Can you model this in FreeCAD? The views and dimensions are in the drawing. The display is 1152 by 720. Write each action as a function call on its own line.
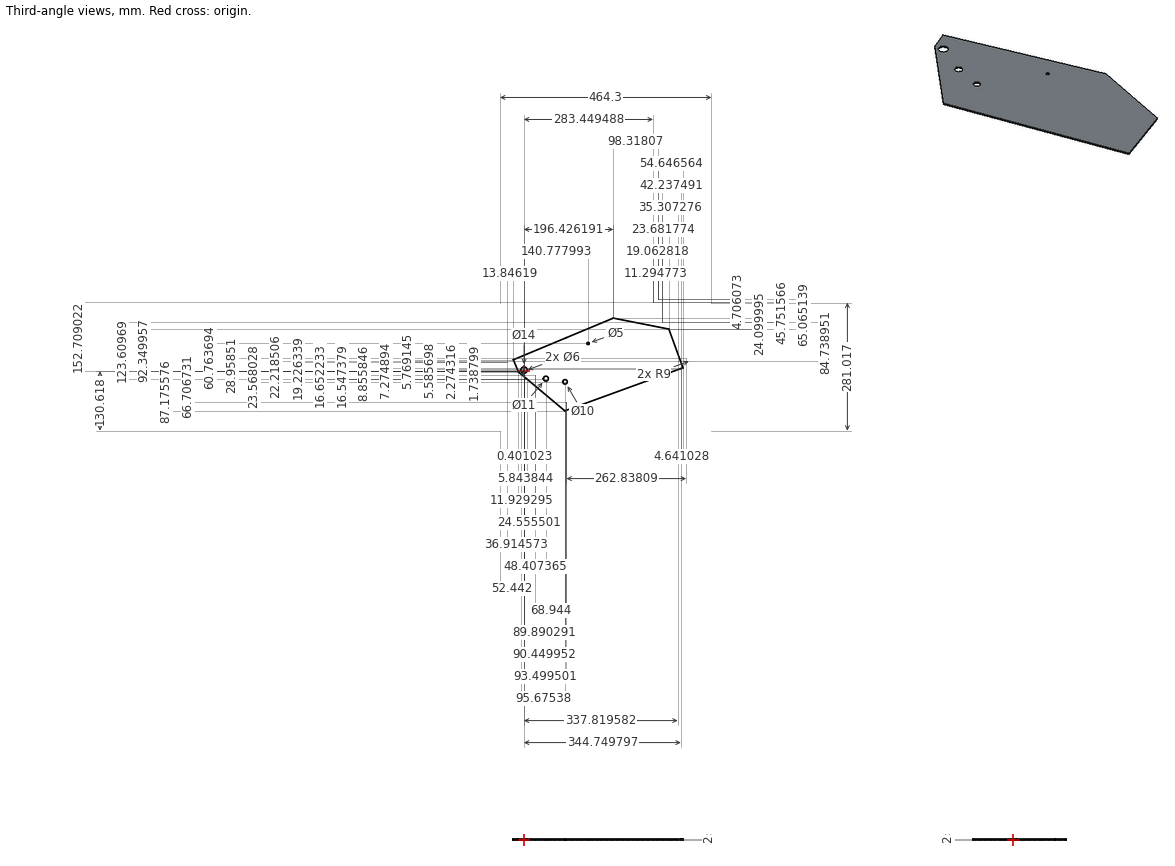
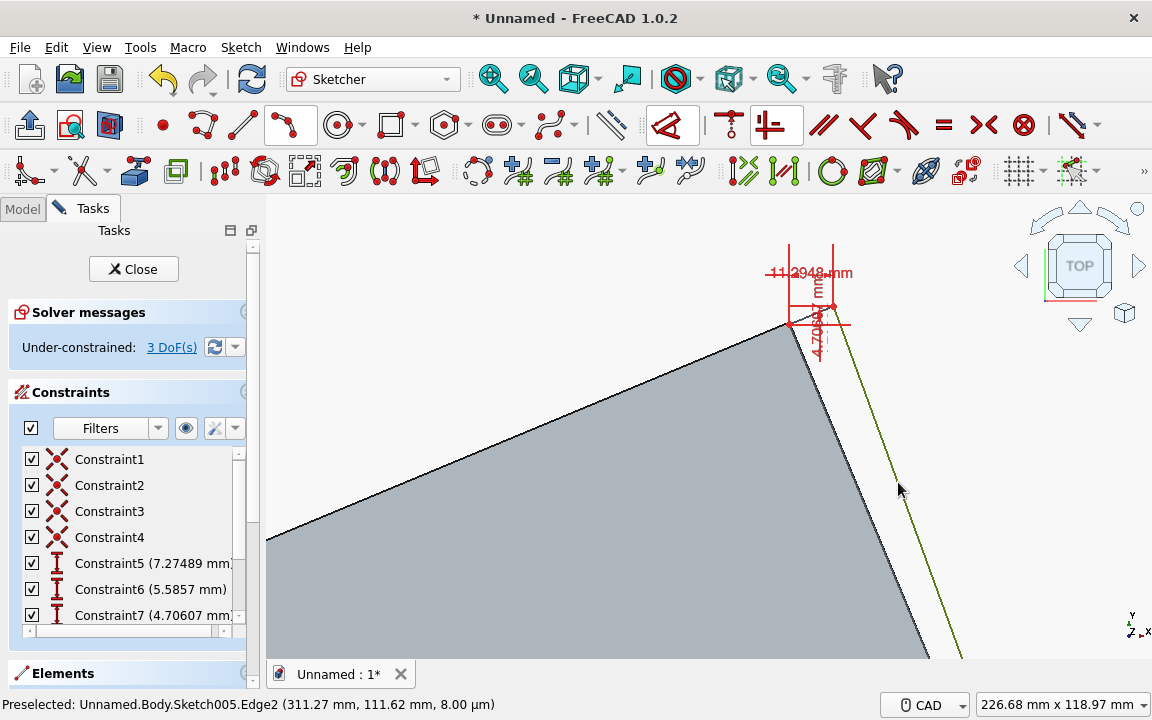
key(l)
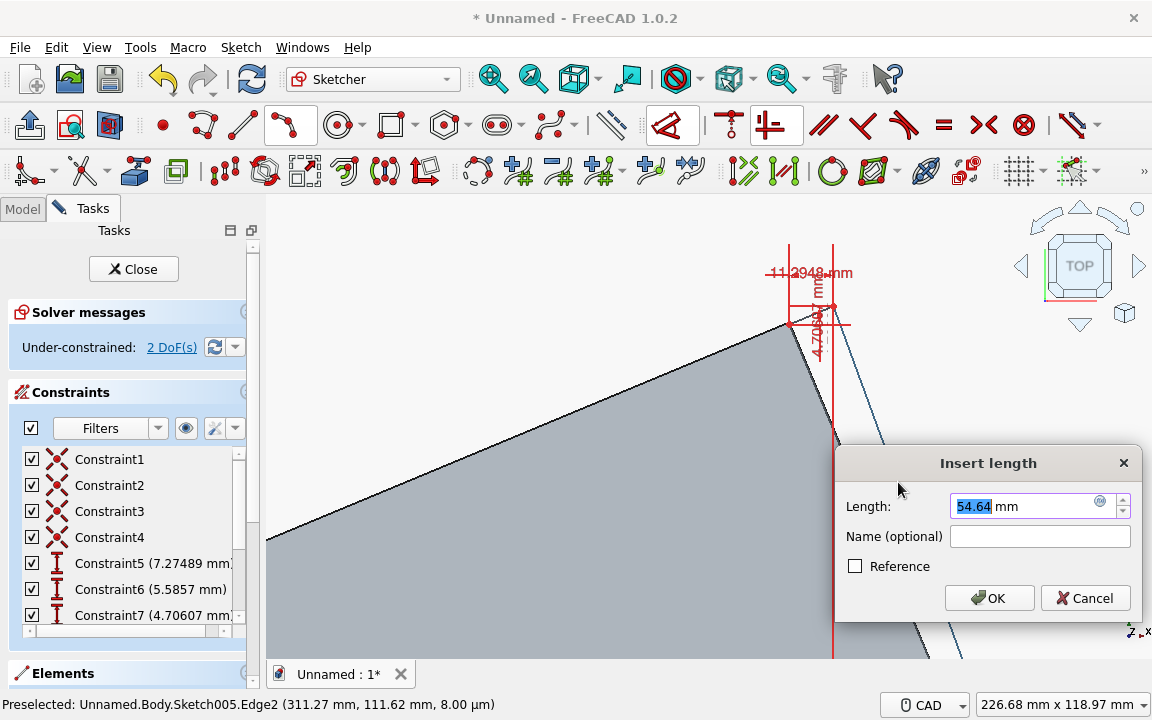
text(54.646564)
key(Return)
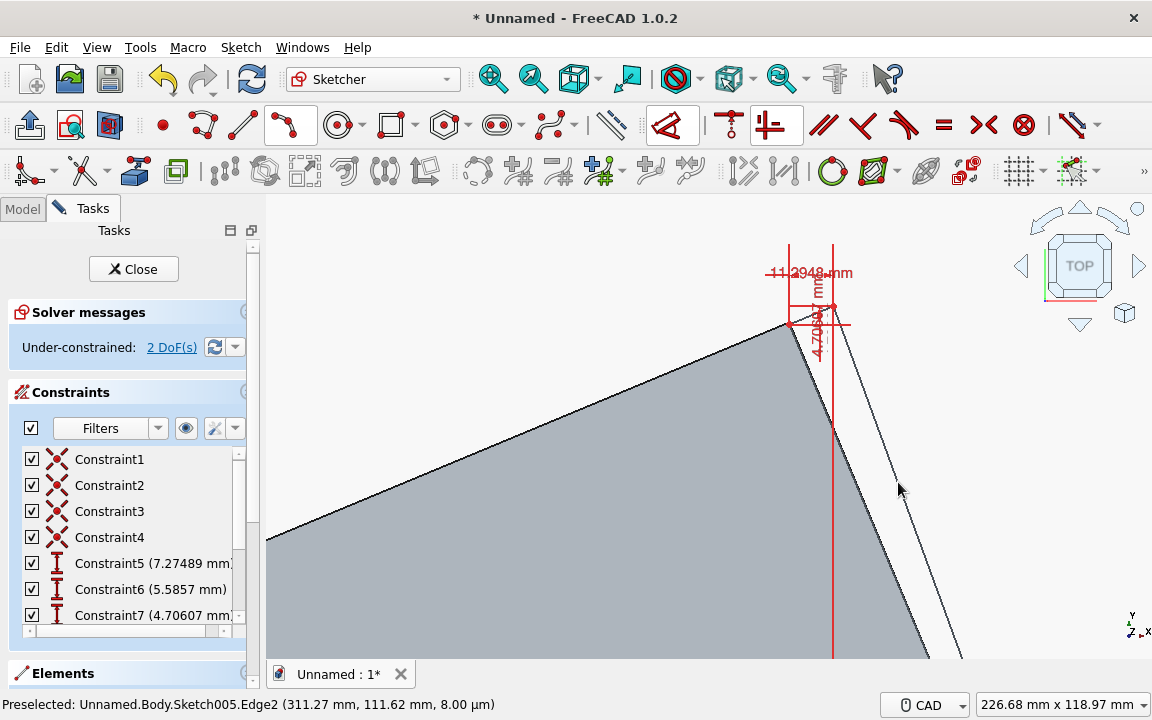
click(789, 325)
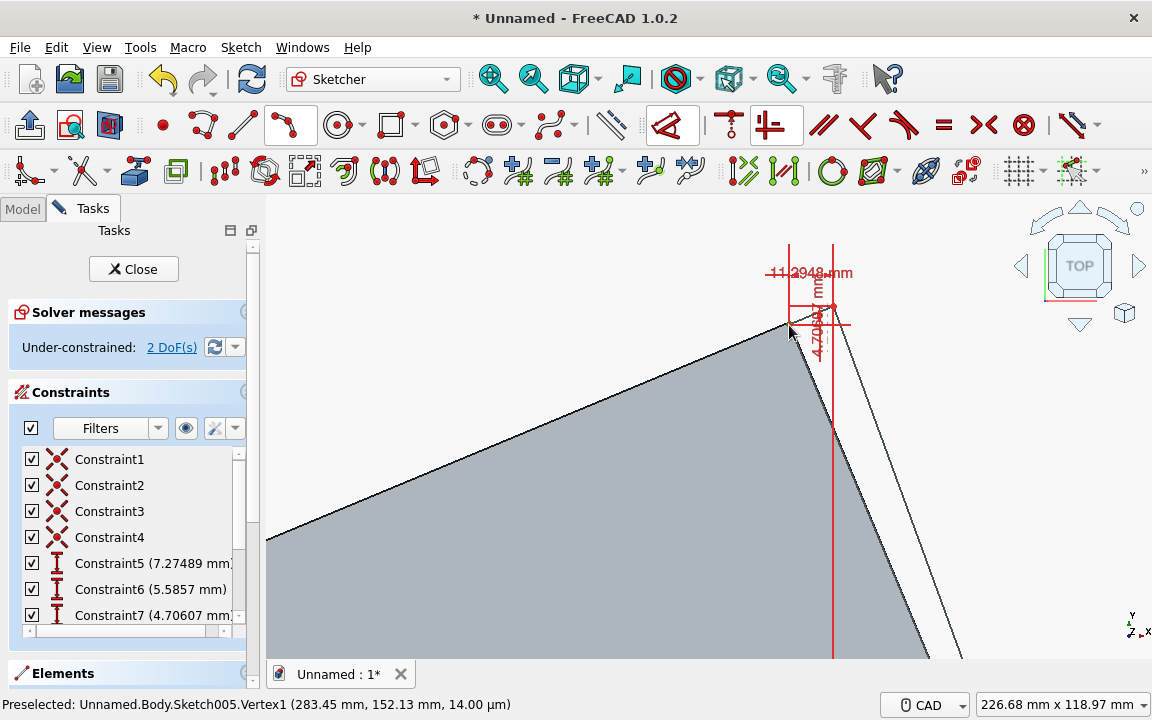
key(l)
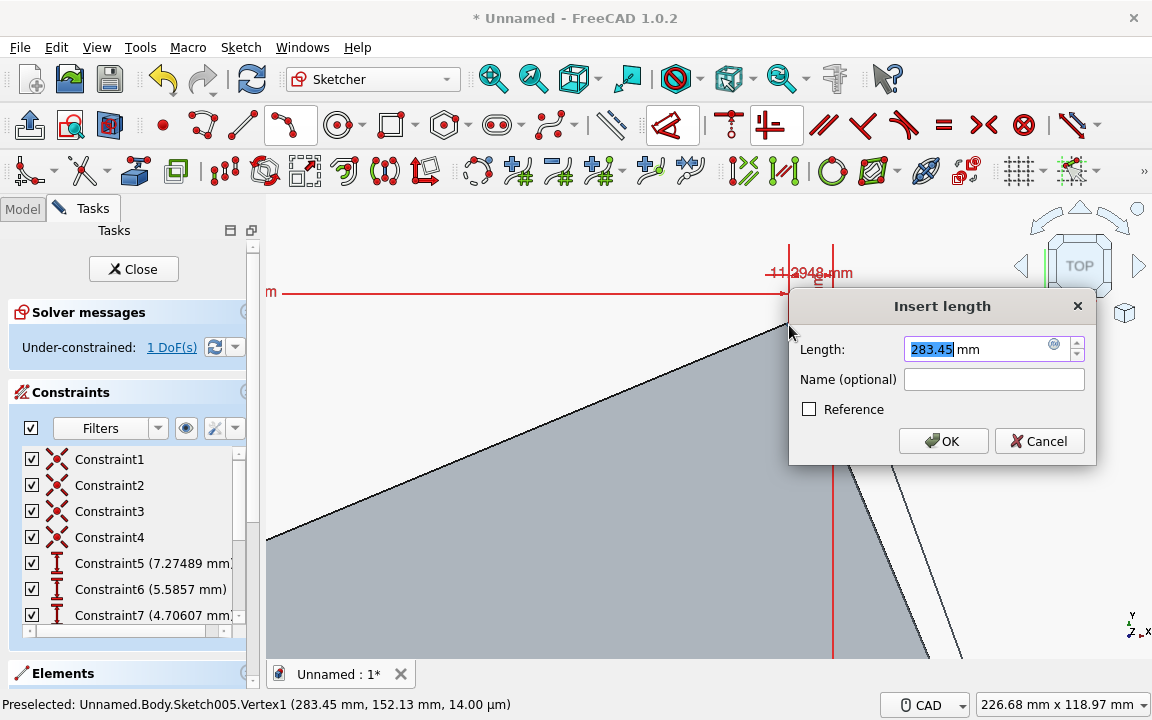
text(283.449488)
key(Return)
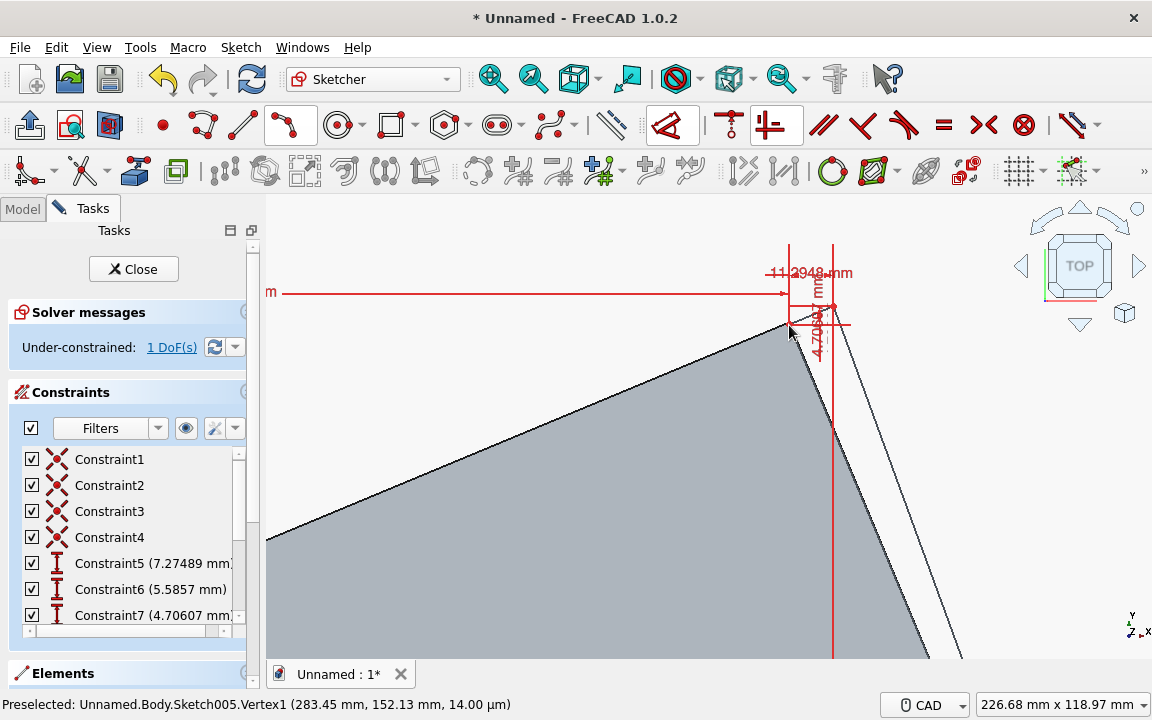
click(789, 325)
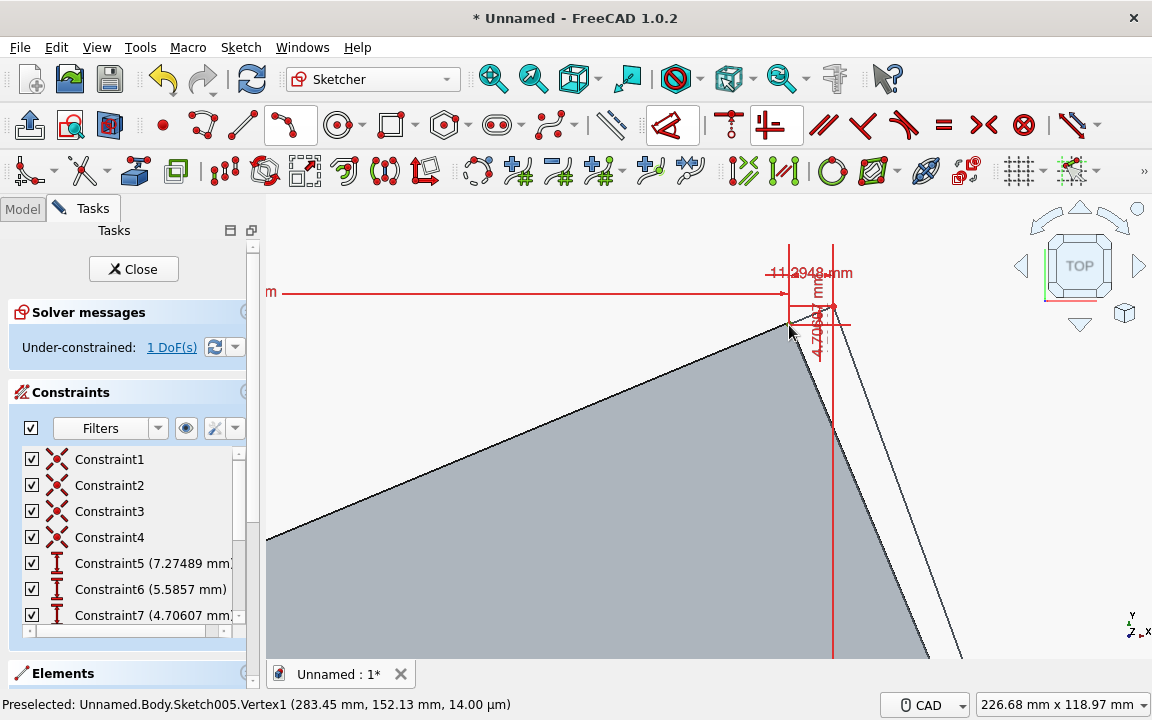
key(i)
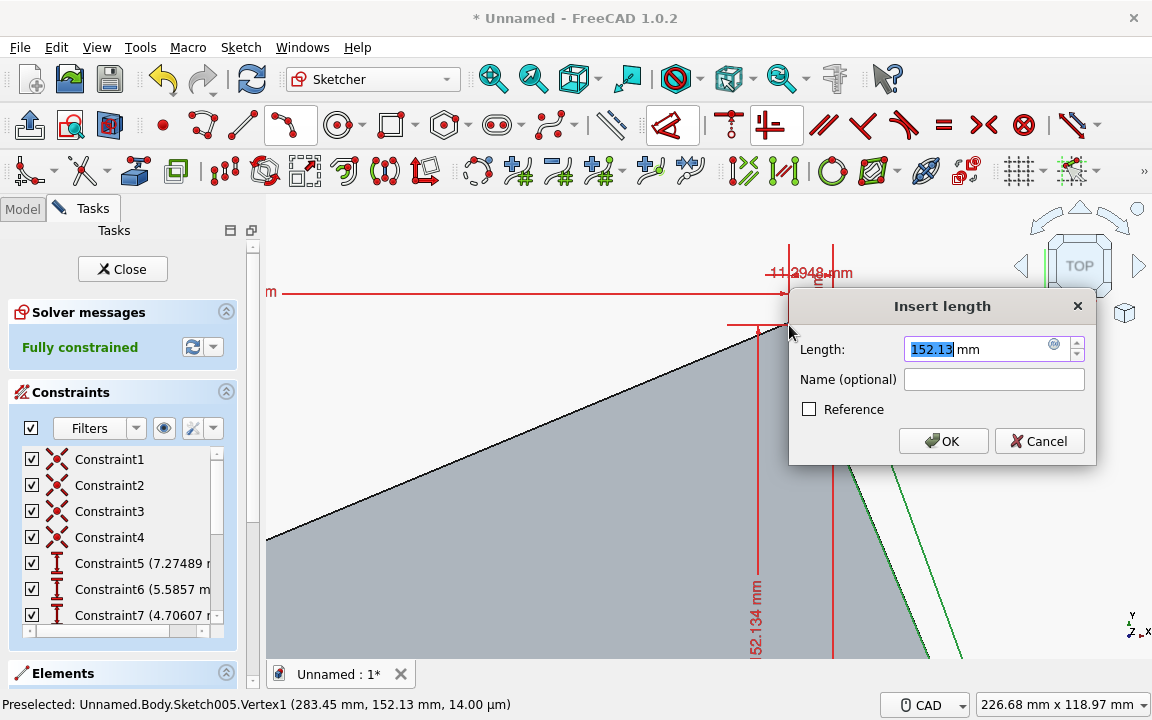
text(152.709022)
key(Return)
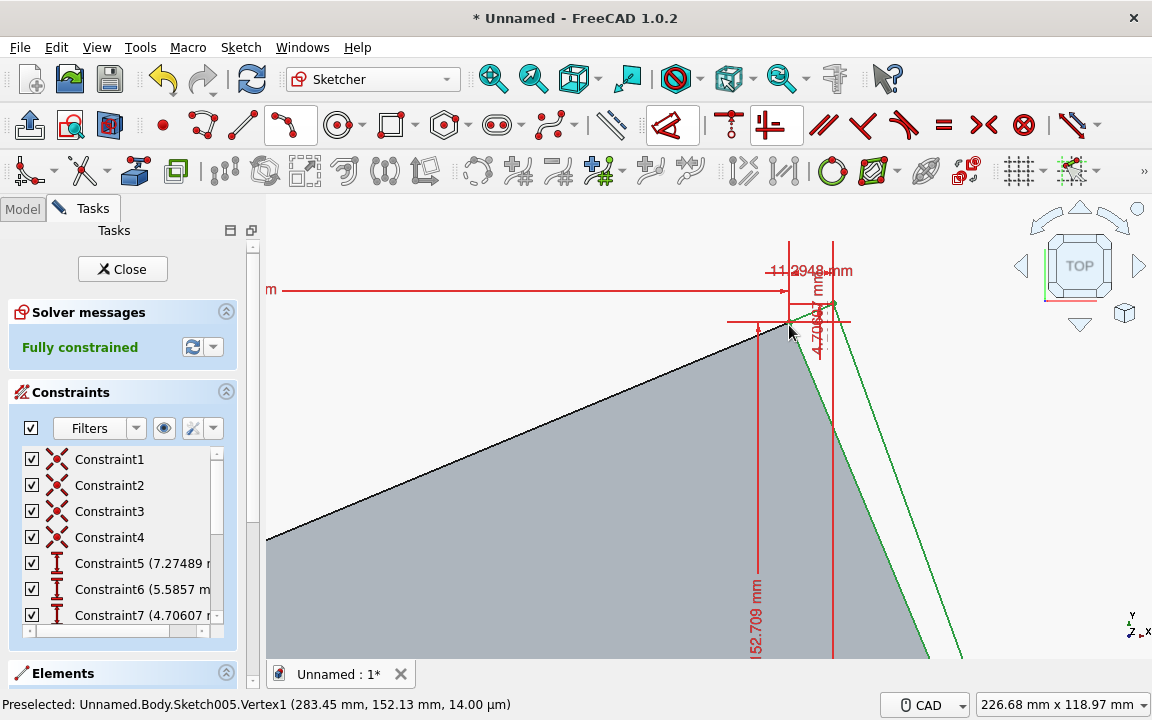
click(123, 269)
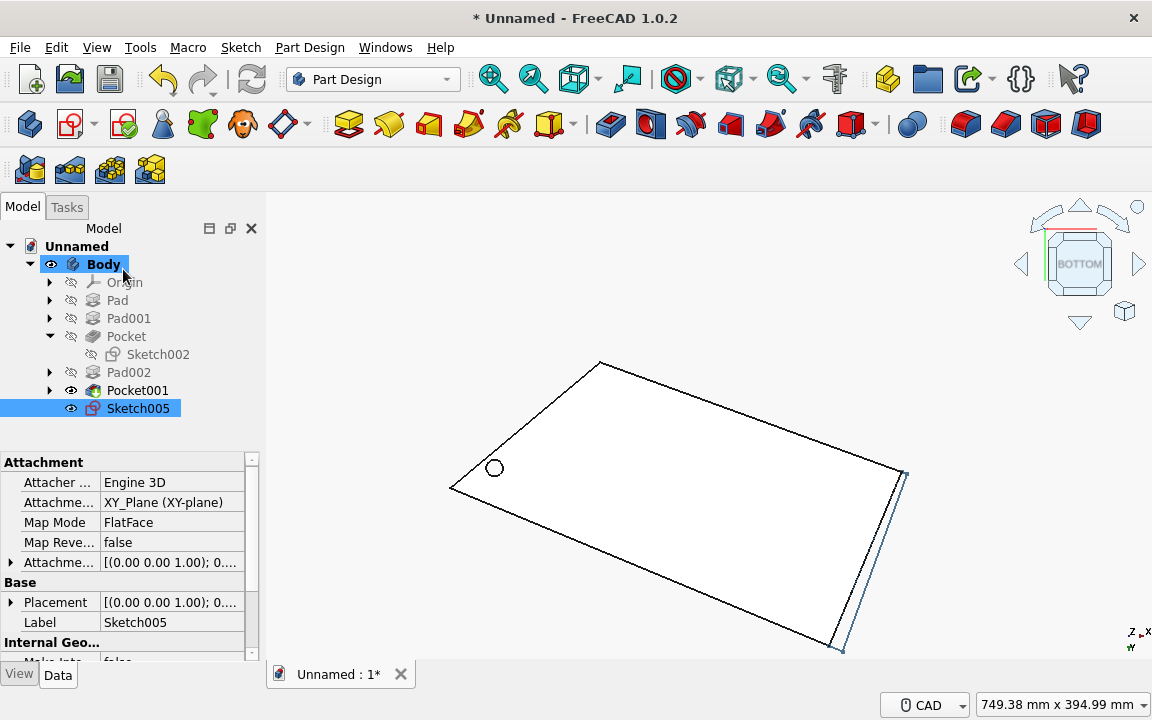
click(350, 124)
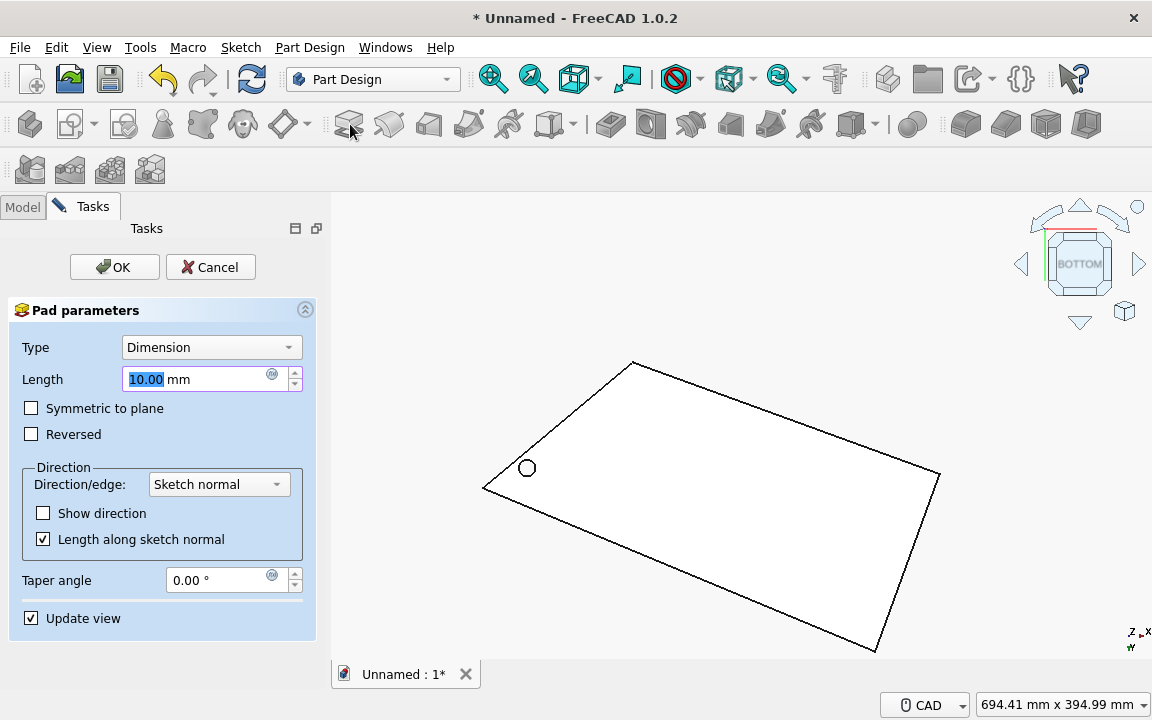
text(2)
key(Tab)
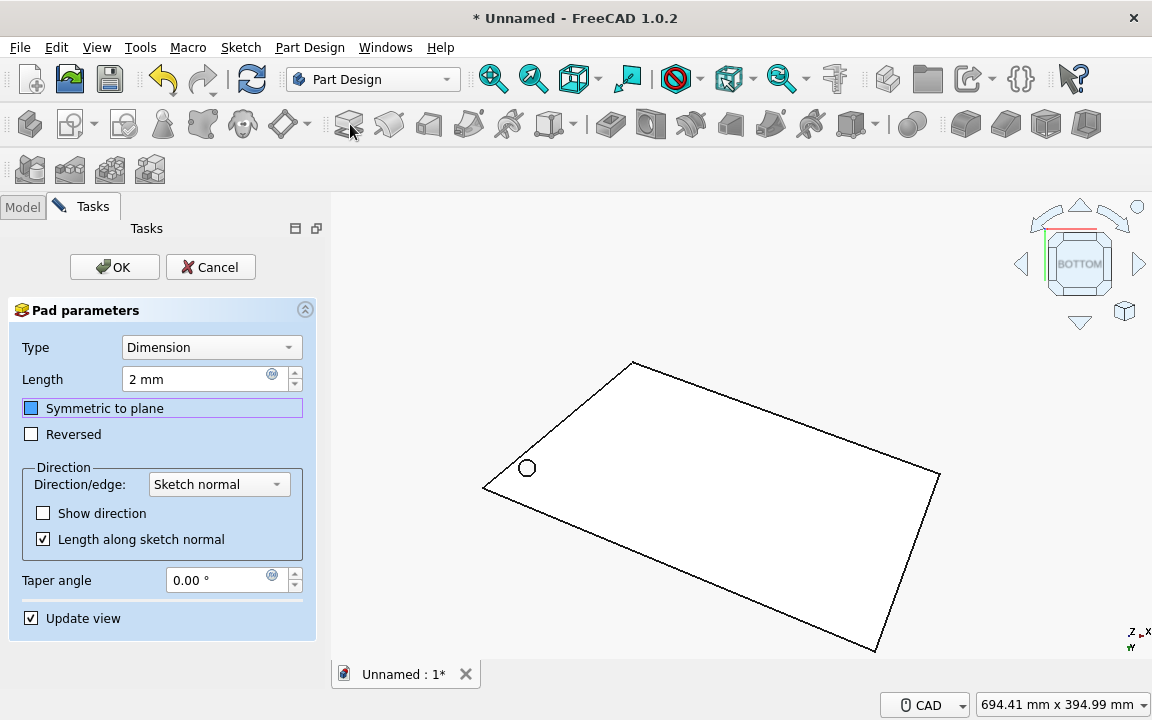
click(115, 267)